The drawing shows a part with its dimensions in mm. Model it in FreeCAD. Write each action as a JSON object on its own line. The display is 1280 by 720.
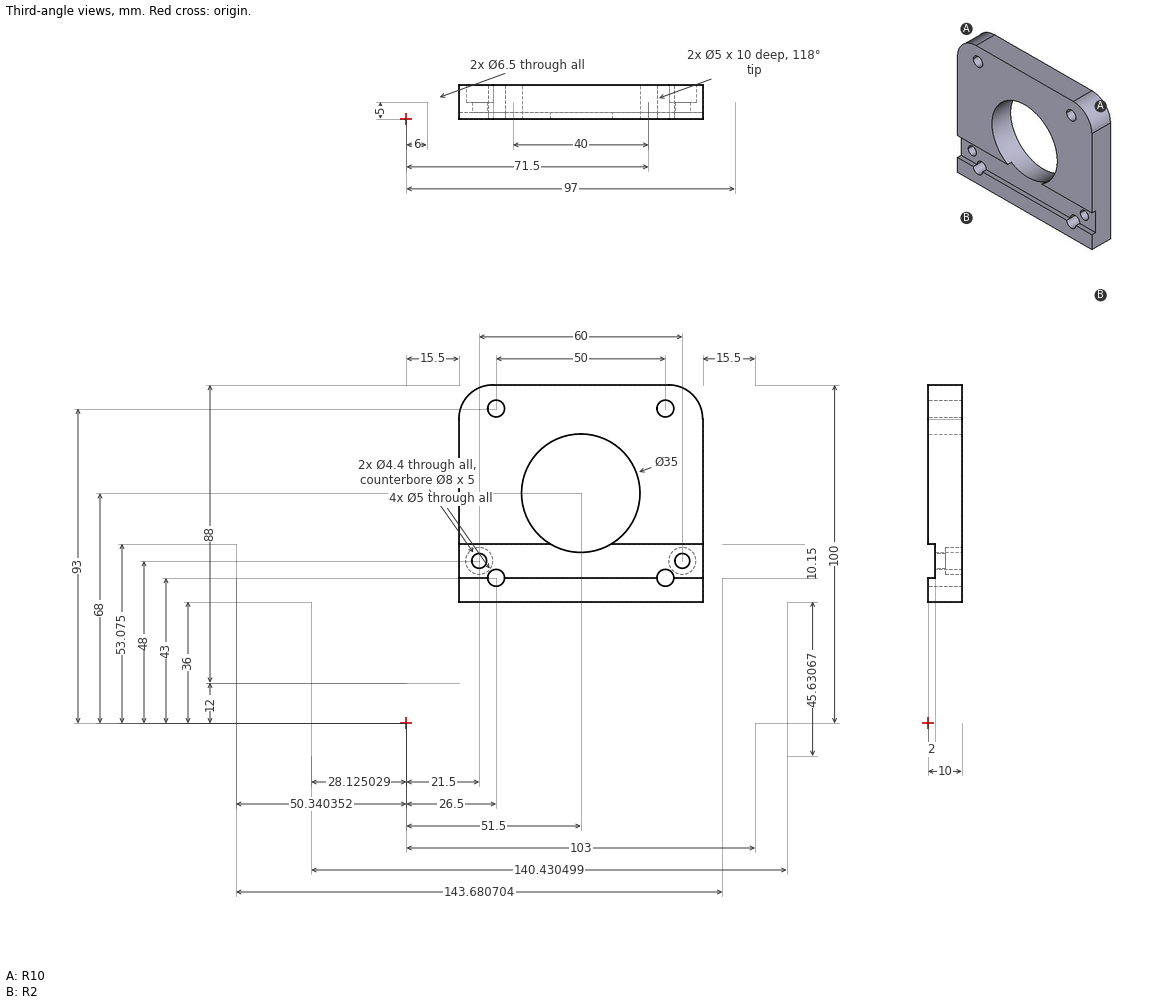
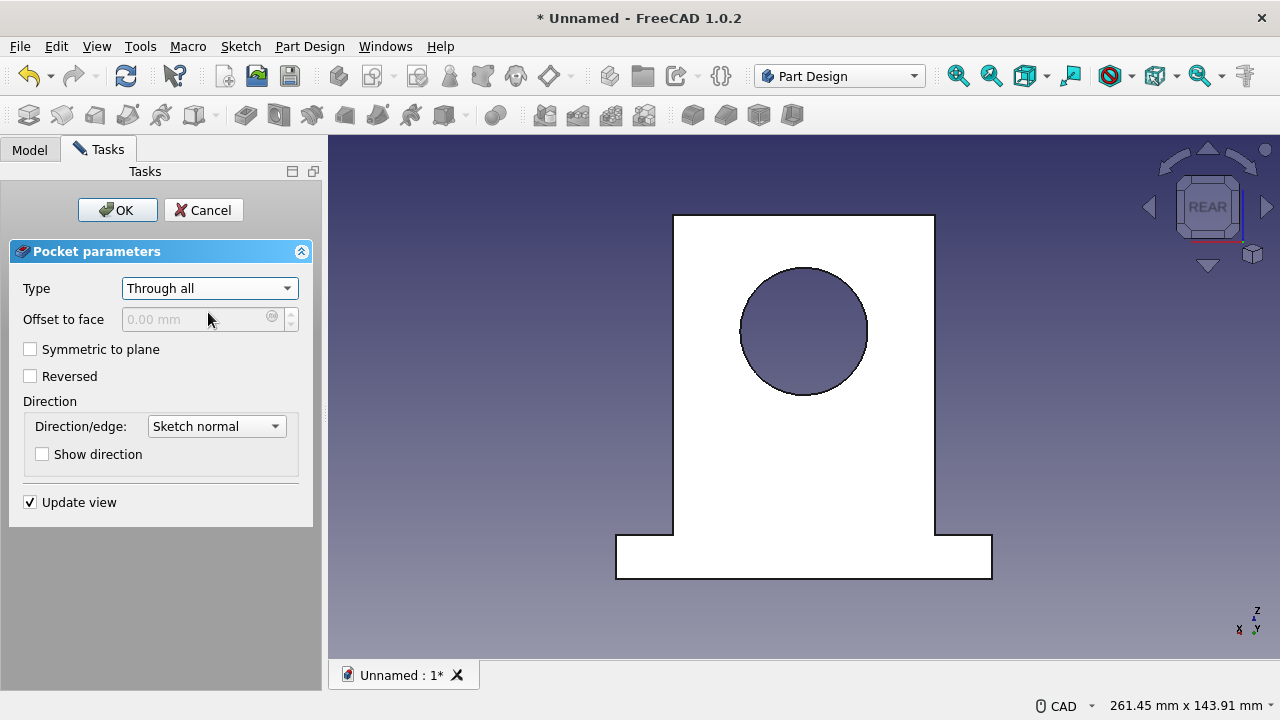
{"action": "left_click", "coordinate": [118, 210]}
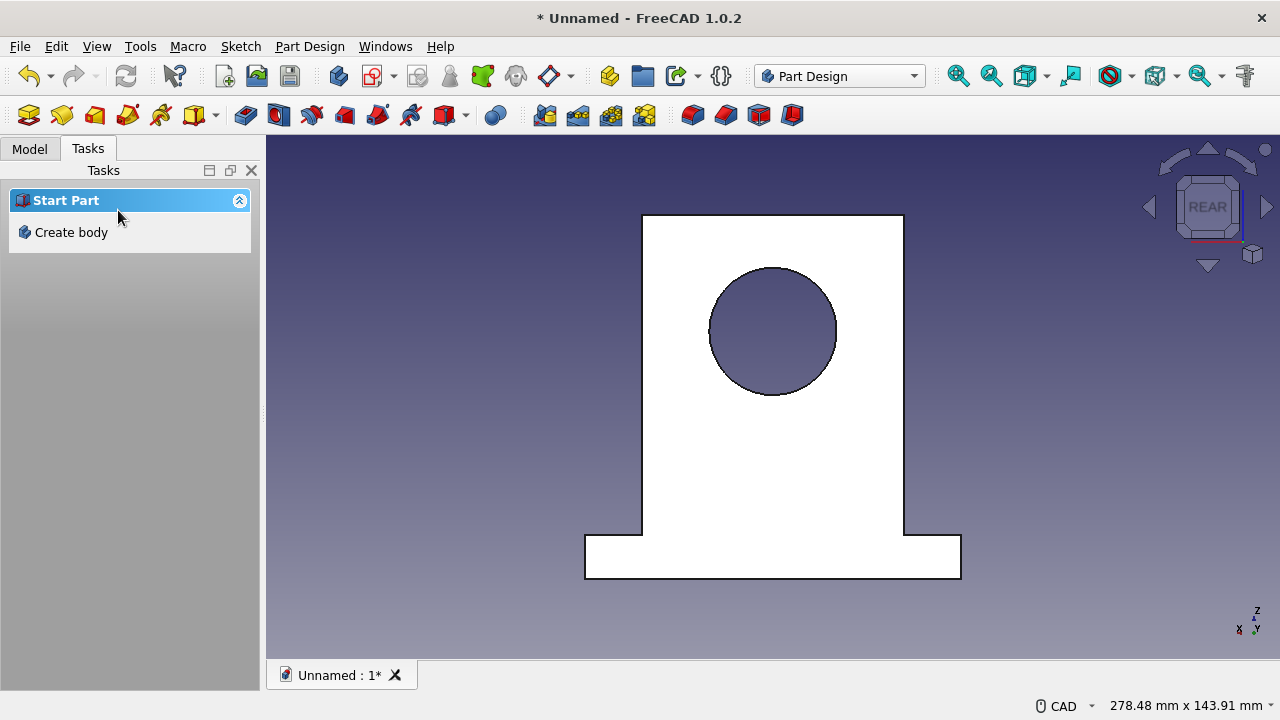
{"action": "key", "text": "0"}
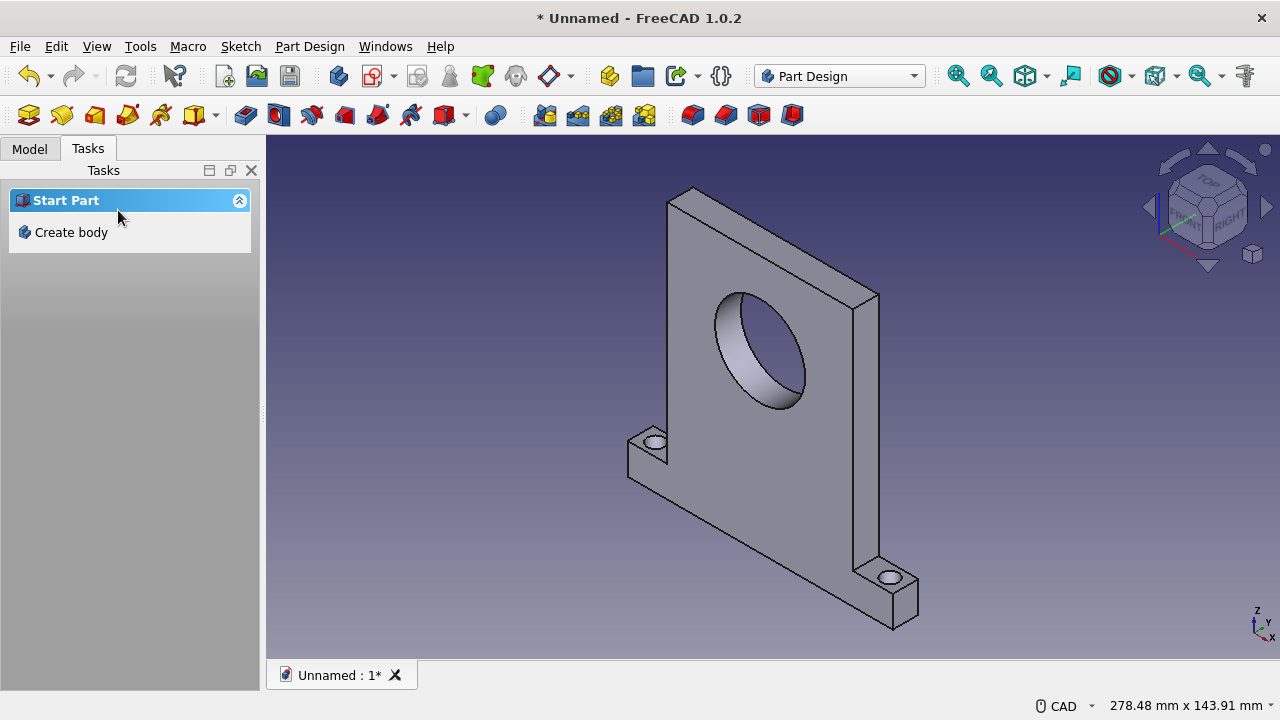
{"action": "left_click", "coordinate": [866, 301]}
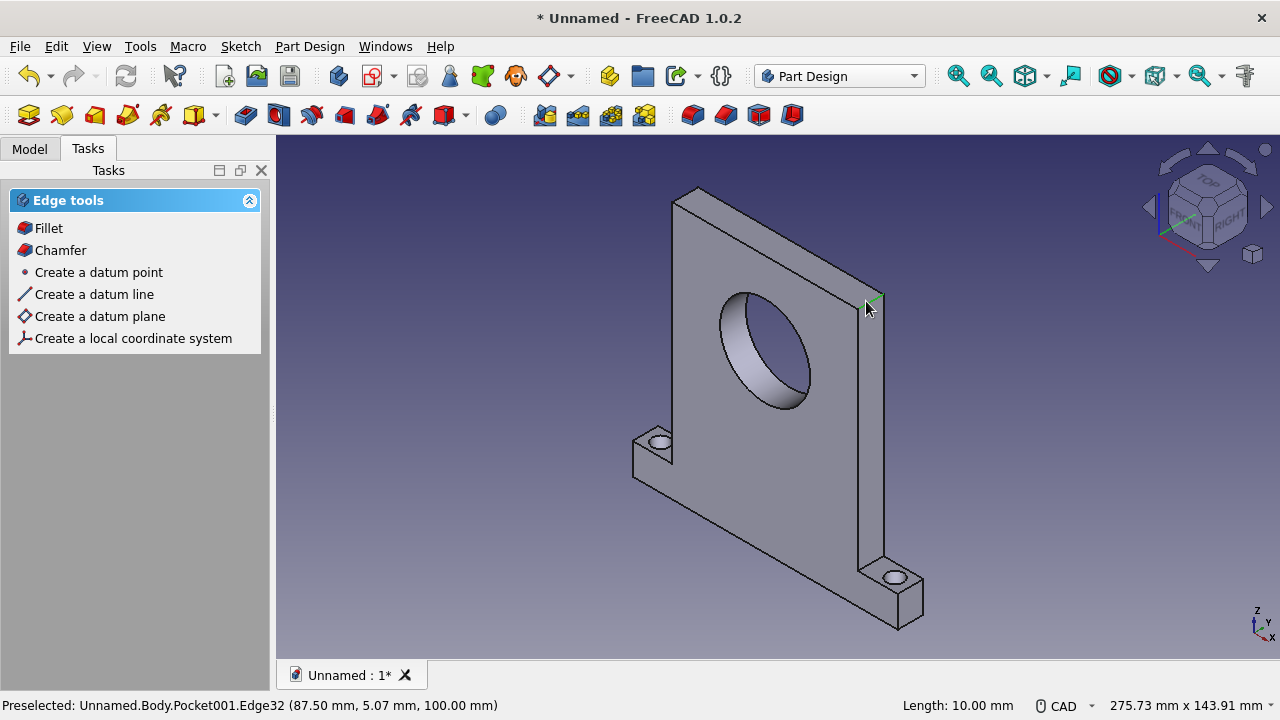
{"action": "key", "text": "2"}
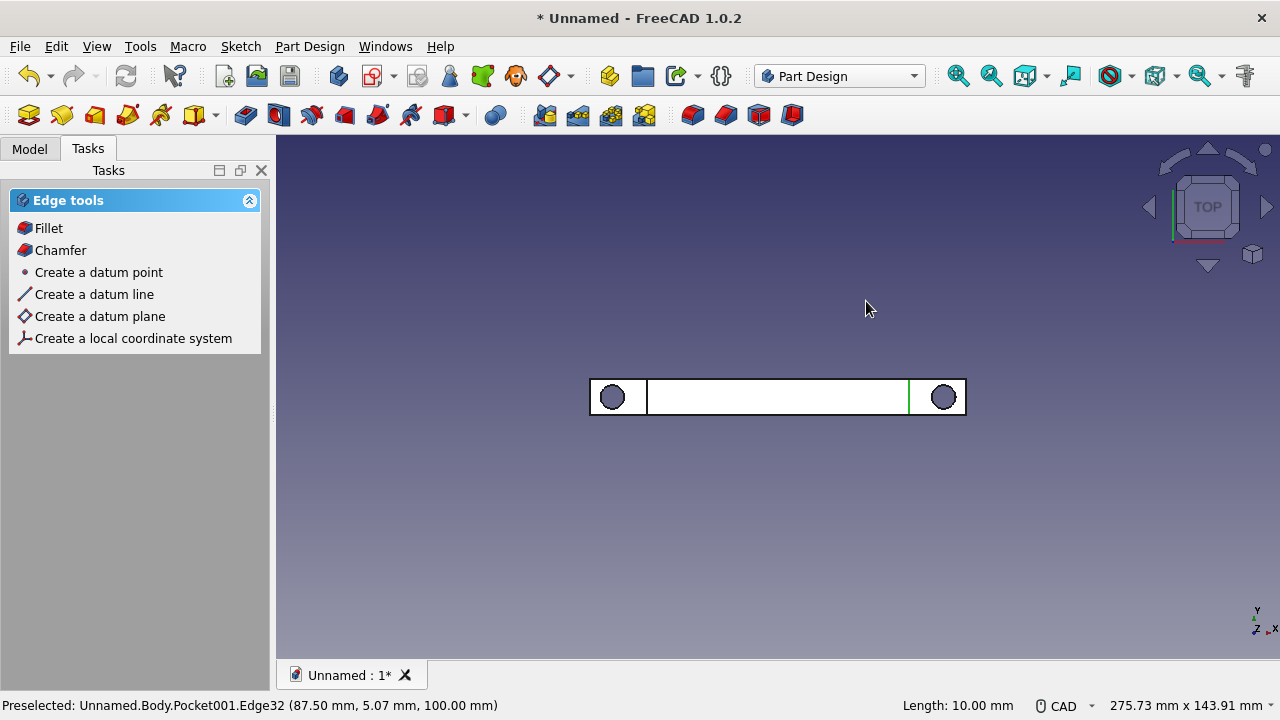
{"action": "left_click", "coordinate": [959, 76]}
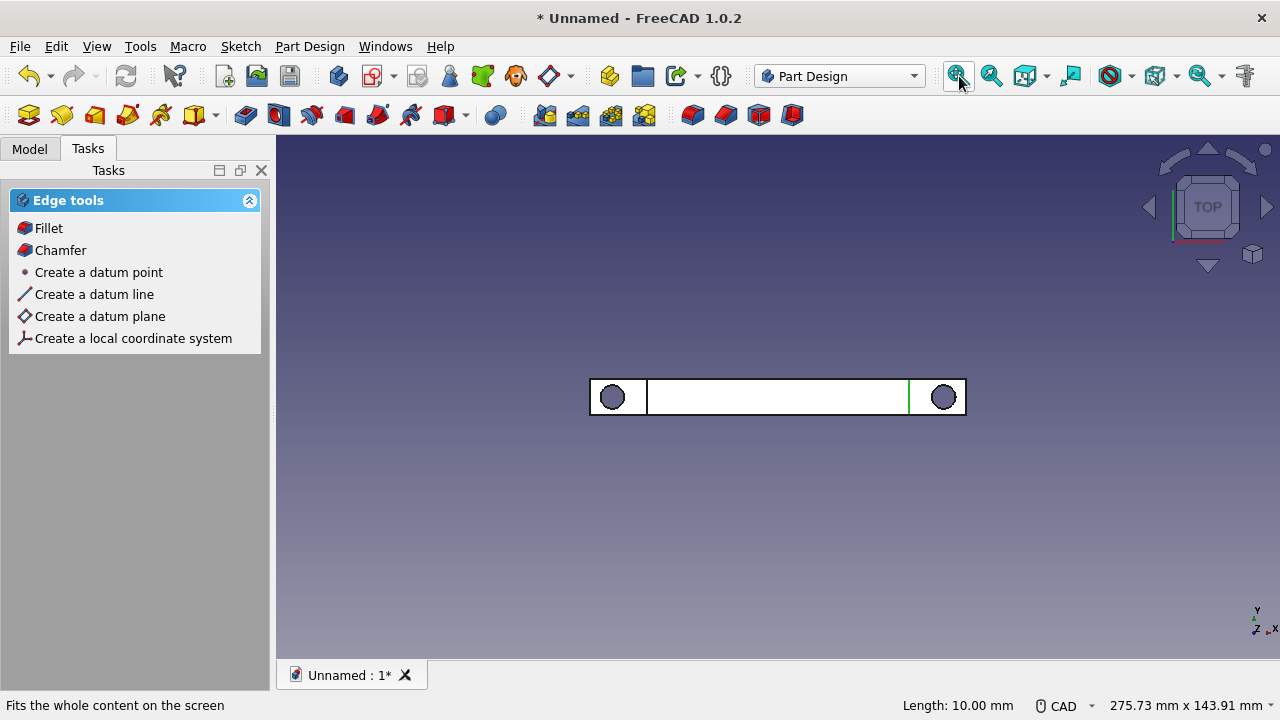
{"action": "left_click", "coordinate": [647, 396], "text": "ctrl"}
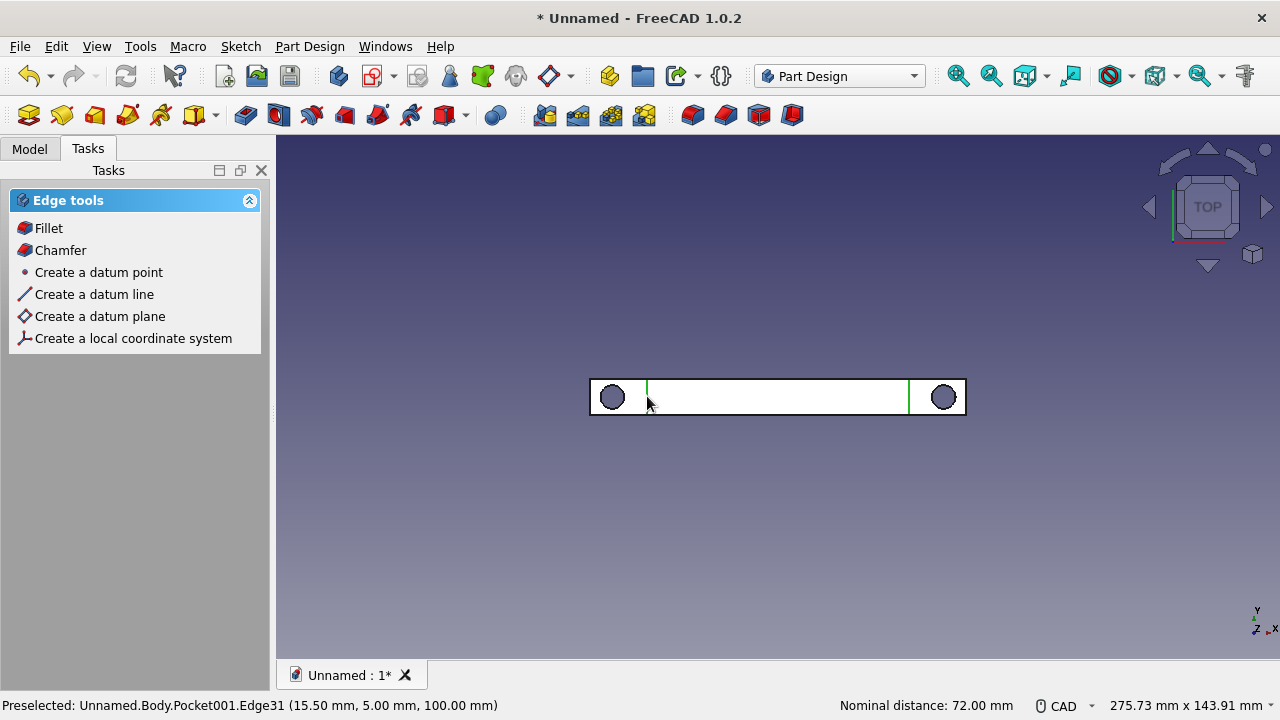
{"action": "left_click", "coordinate": [693, 116]}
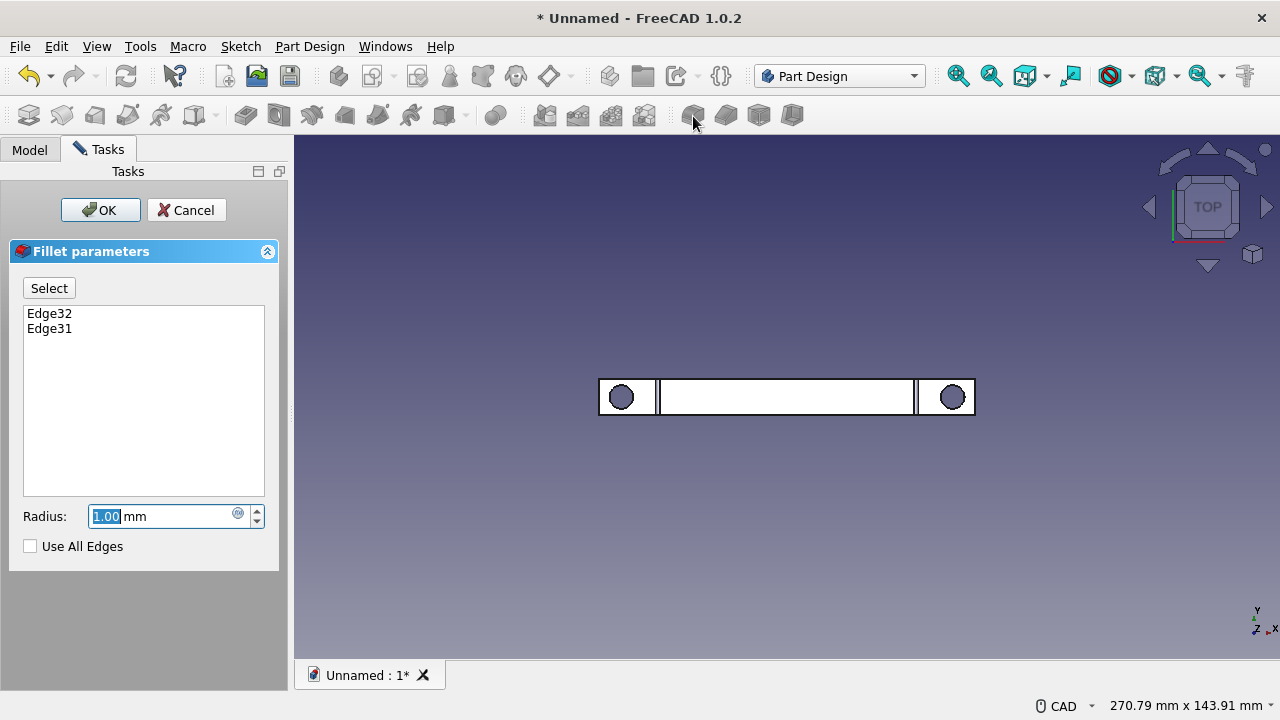
{"action": "type", "text": "10"}
{"action": "key", "text": "Tab"}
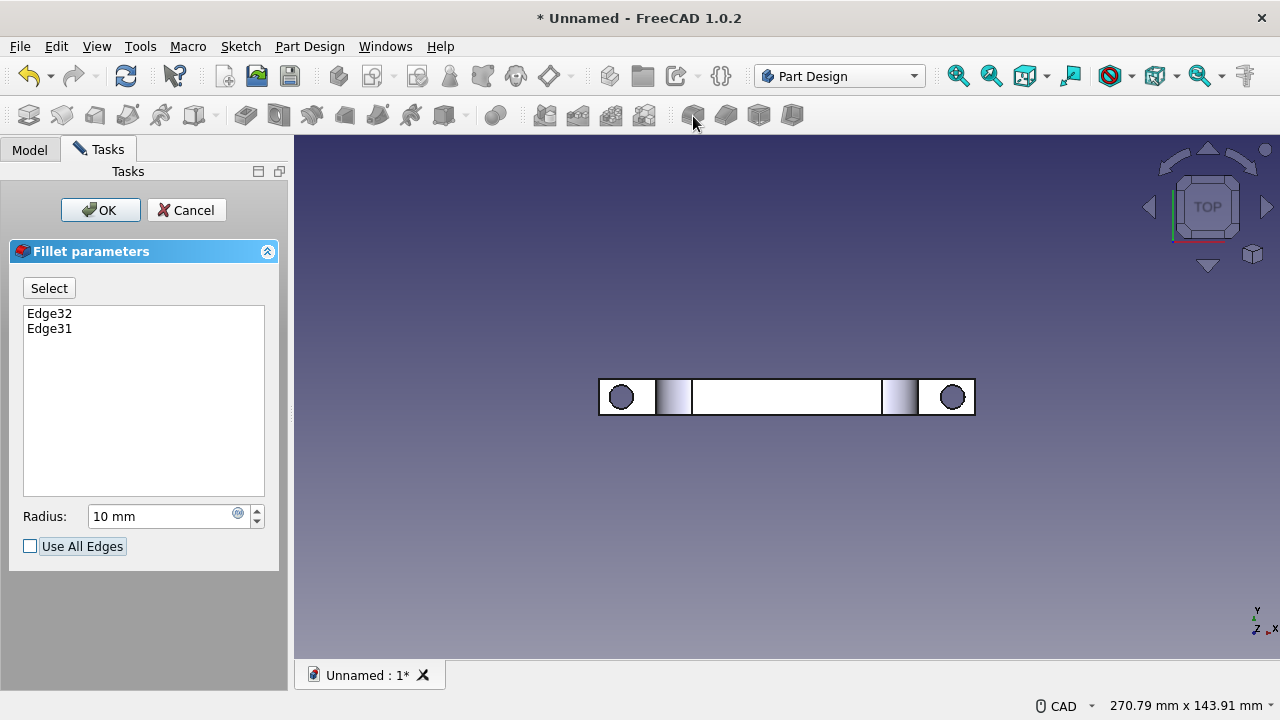
{"action": "left_click", "coordinate": [101, 210]}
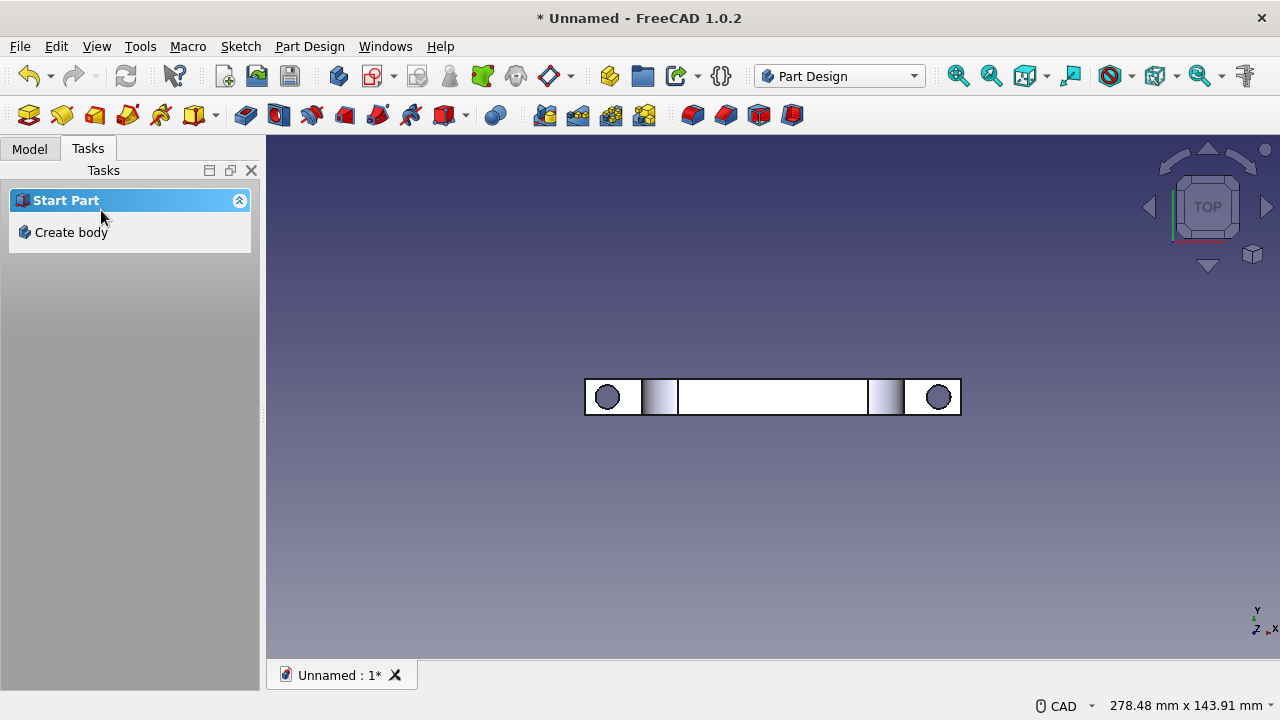
{"action": "left_click", "coordinate": [959, 76]}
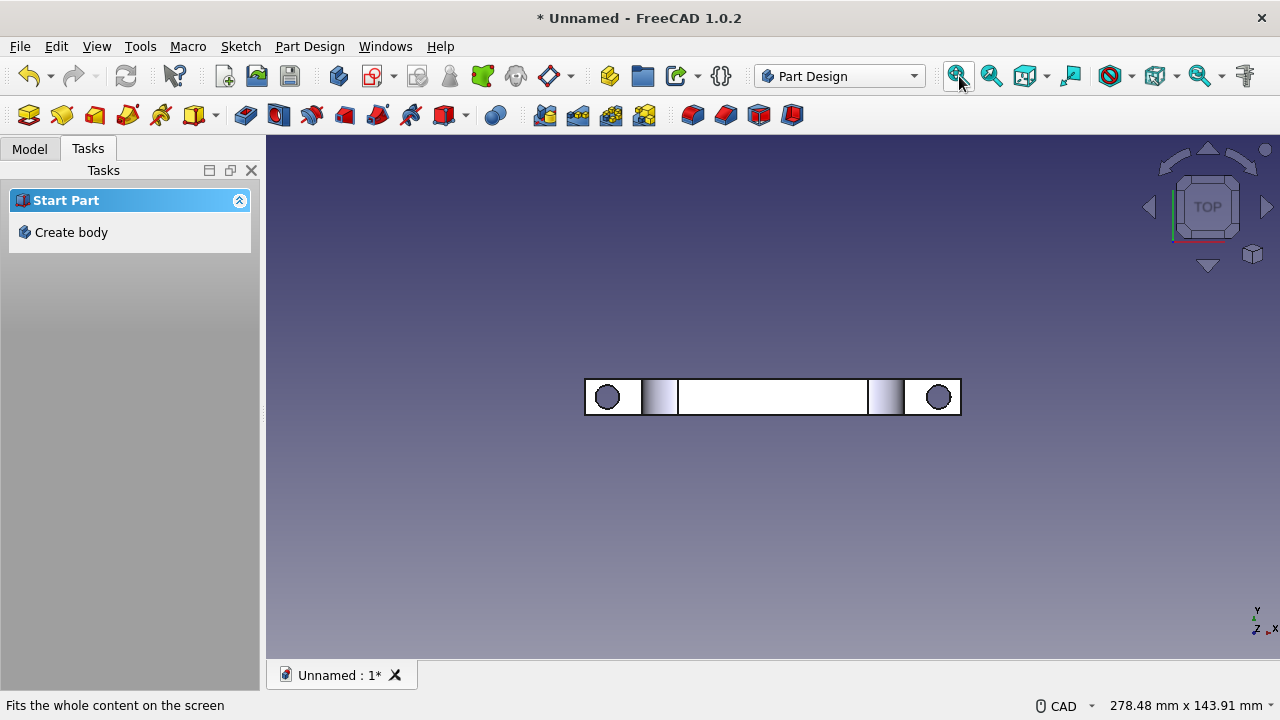
{"action": "left_click", "coordinate": [372, 76]}